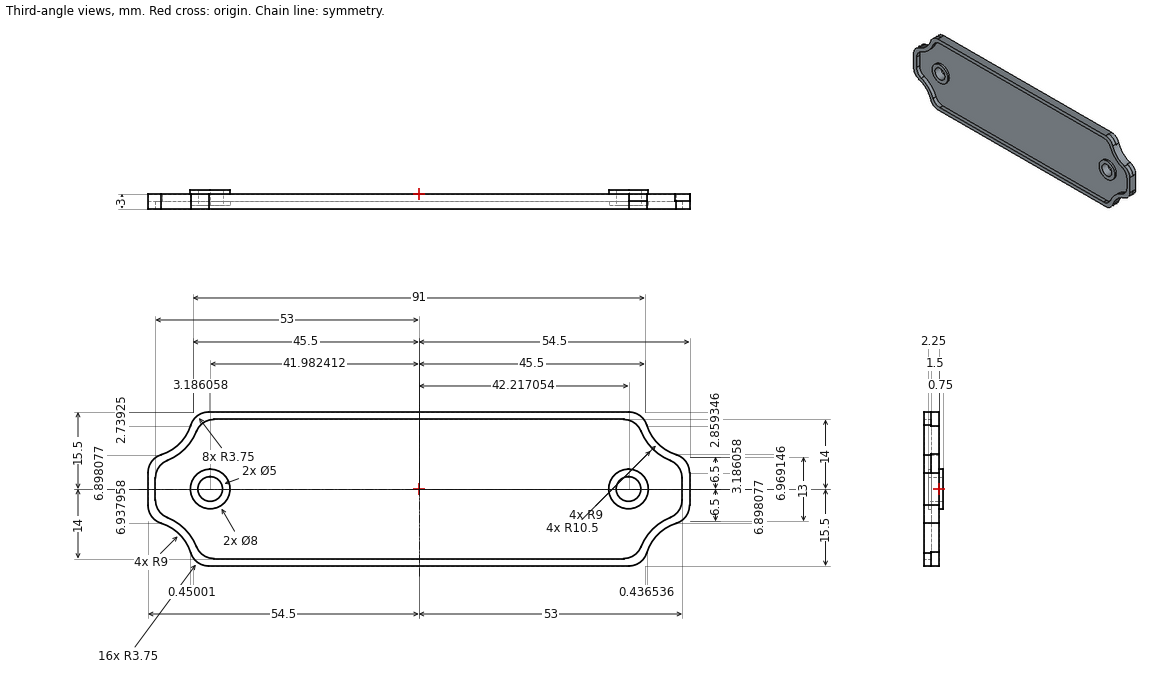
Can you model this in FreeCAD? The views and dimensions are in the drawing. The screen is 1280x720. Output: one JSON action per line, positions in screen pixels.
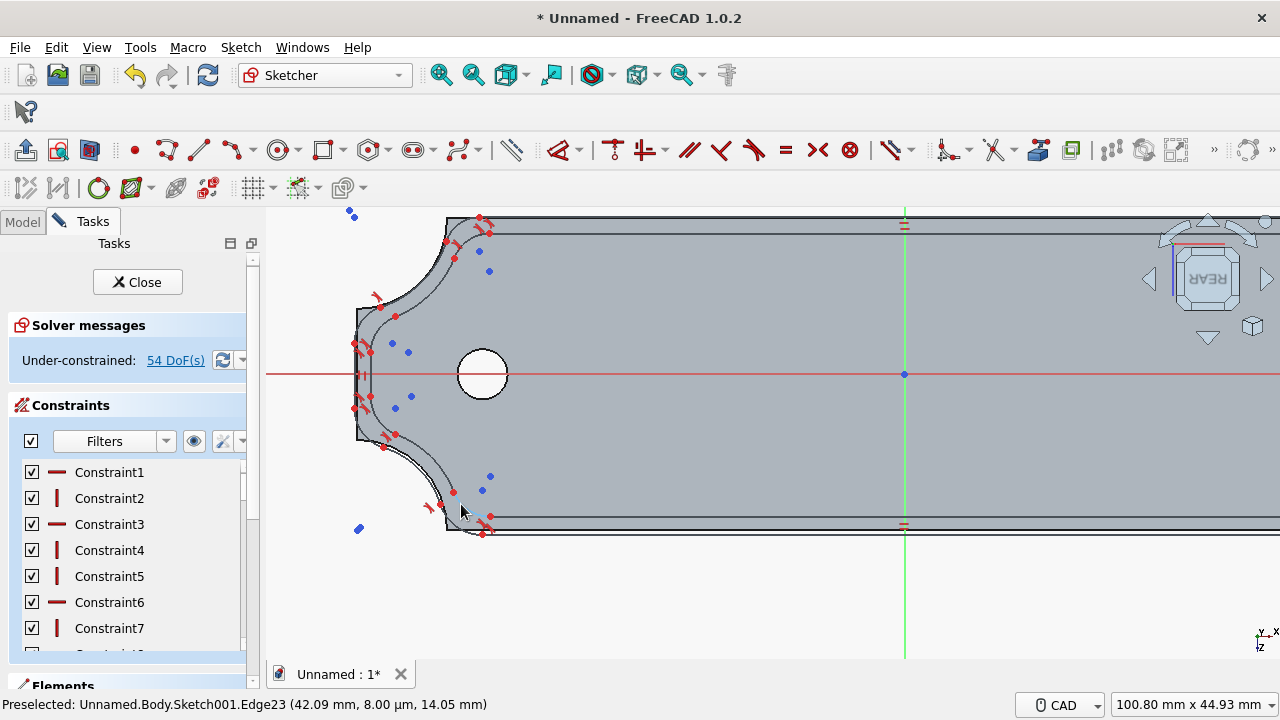
{"action": "left_click", "coordinate": [462, 504]}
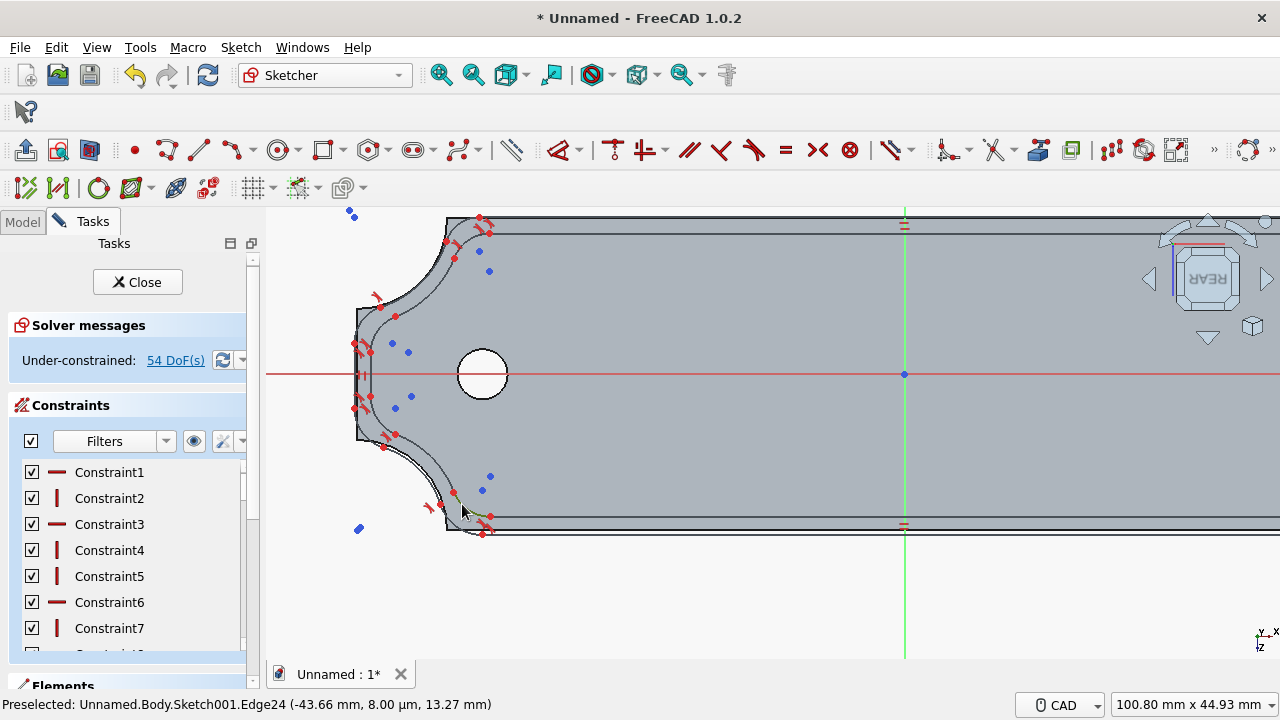
{"action": "left_click", "coordinate": [442, 470]}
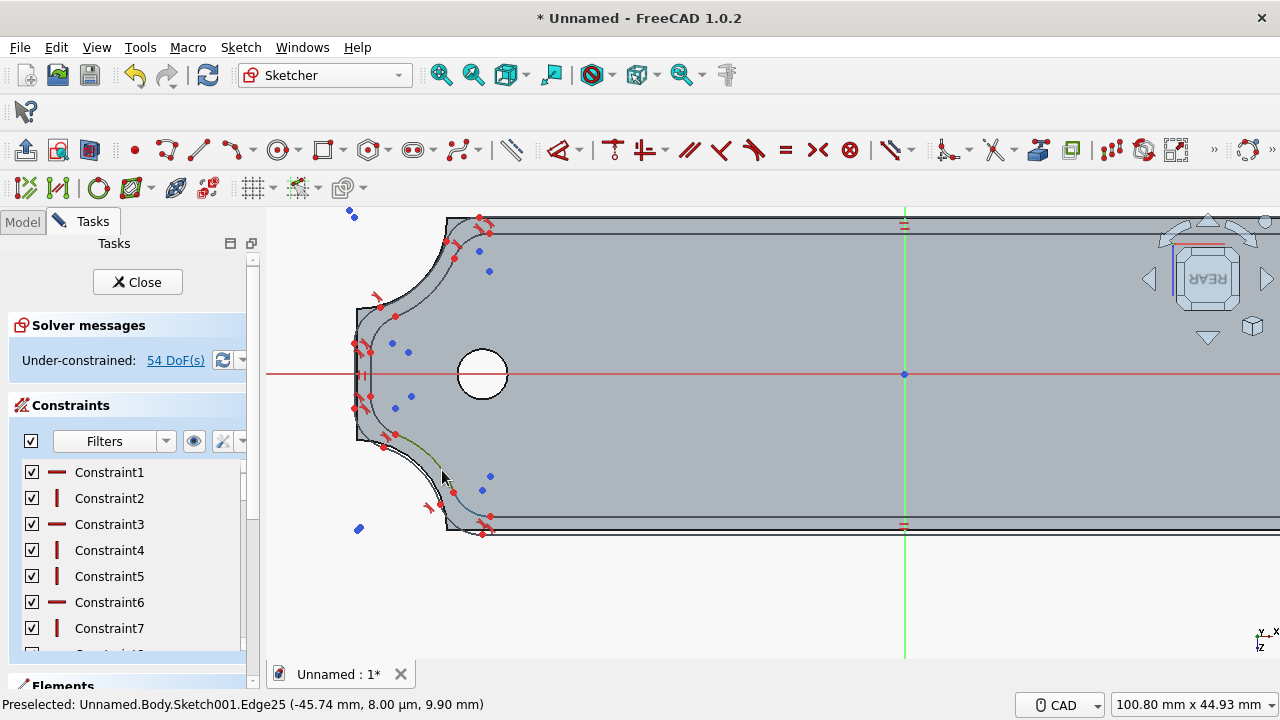
{"action": "left_click", "coordinate": [754, 150]}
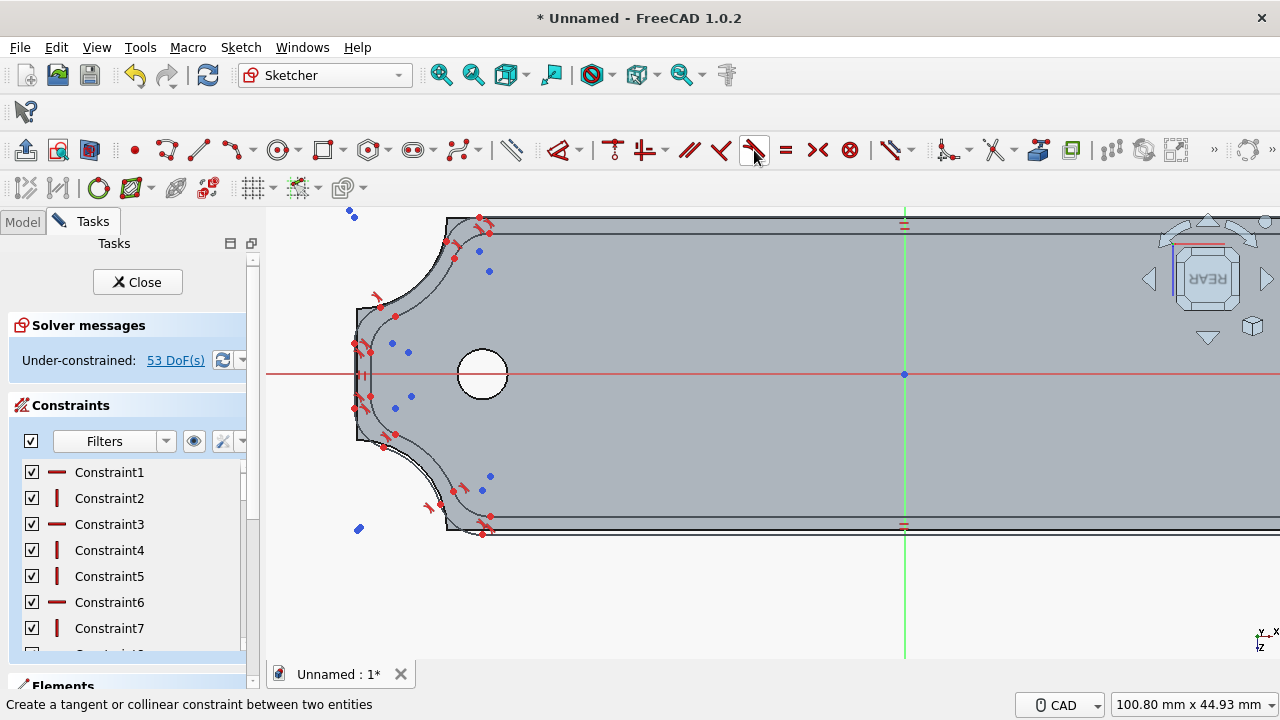
{"action": "left_click", "coordinate": [442, 469]}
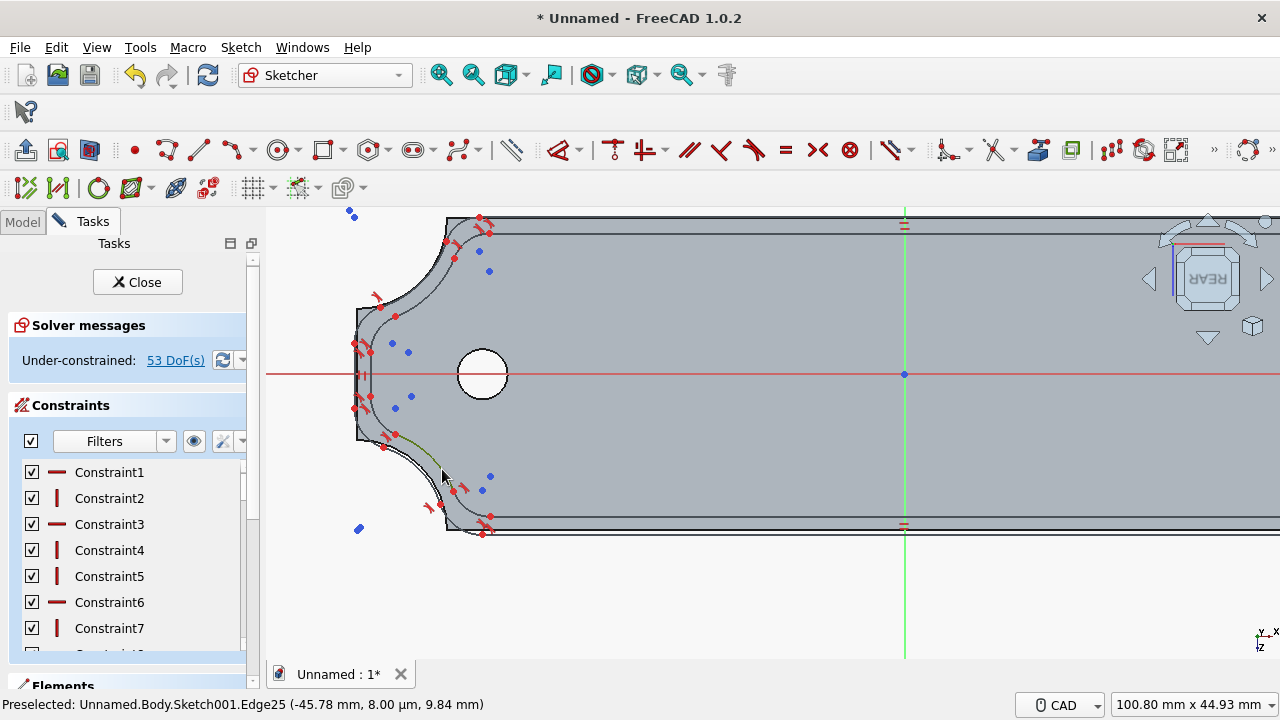
{"action": "left_click", "coordinate": [373, 410]}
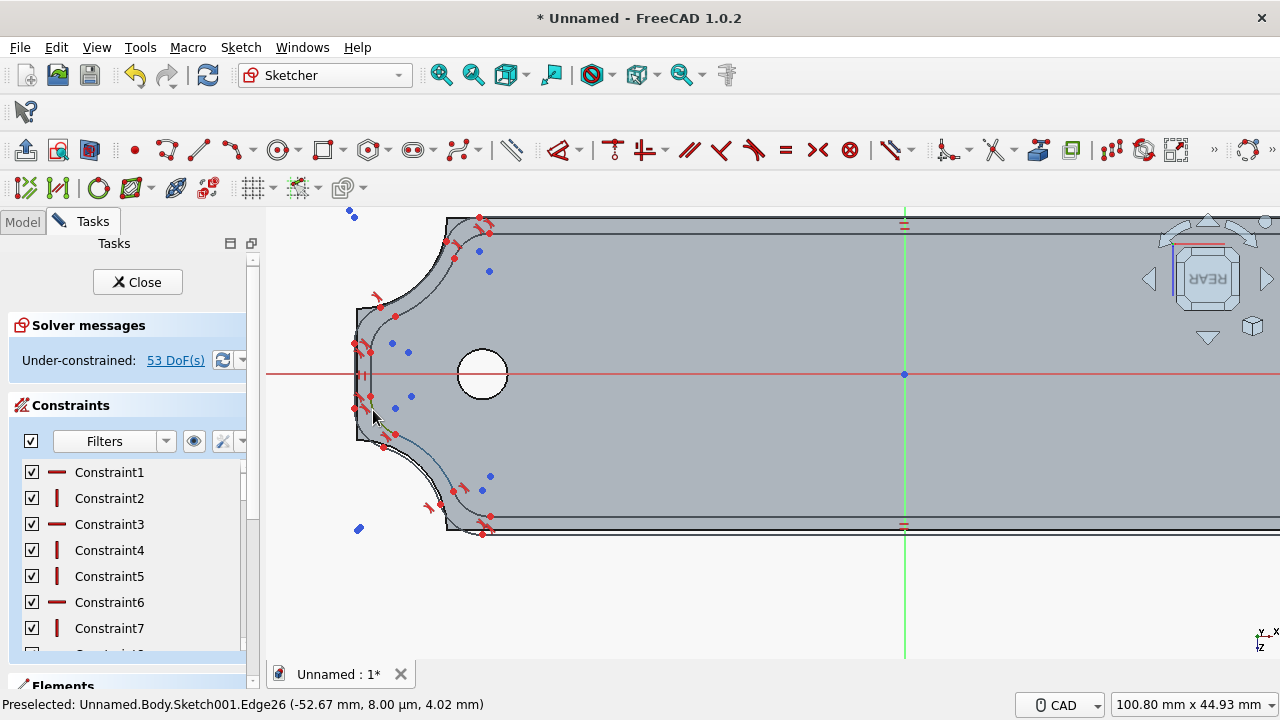
{"action": "left_click", "coordinate": [754, 150]}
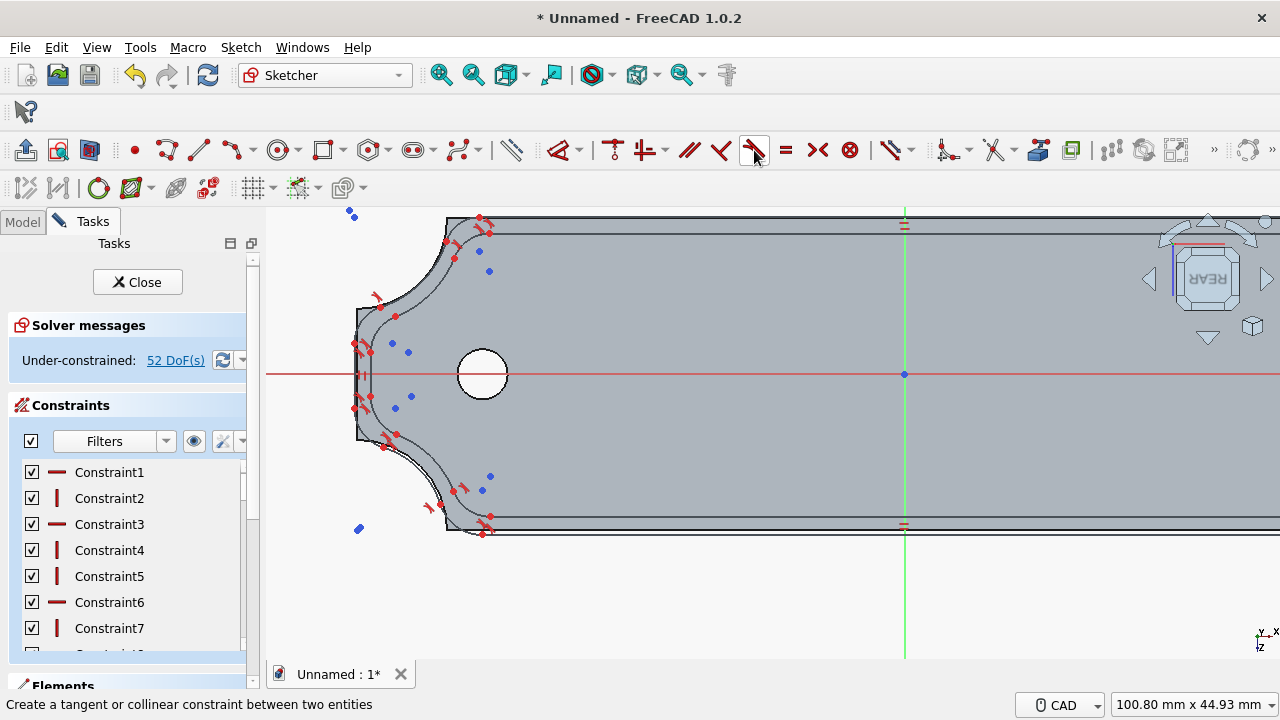
{"action": "left_click", "coordinate": [384, 324]}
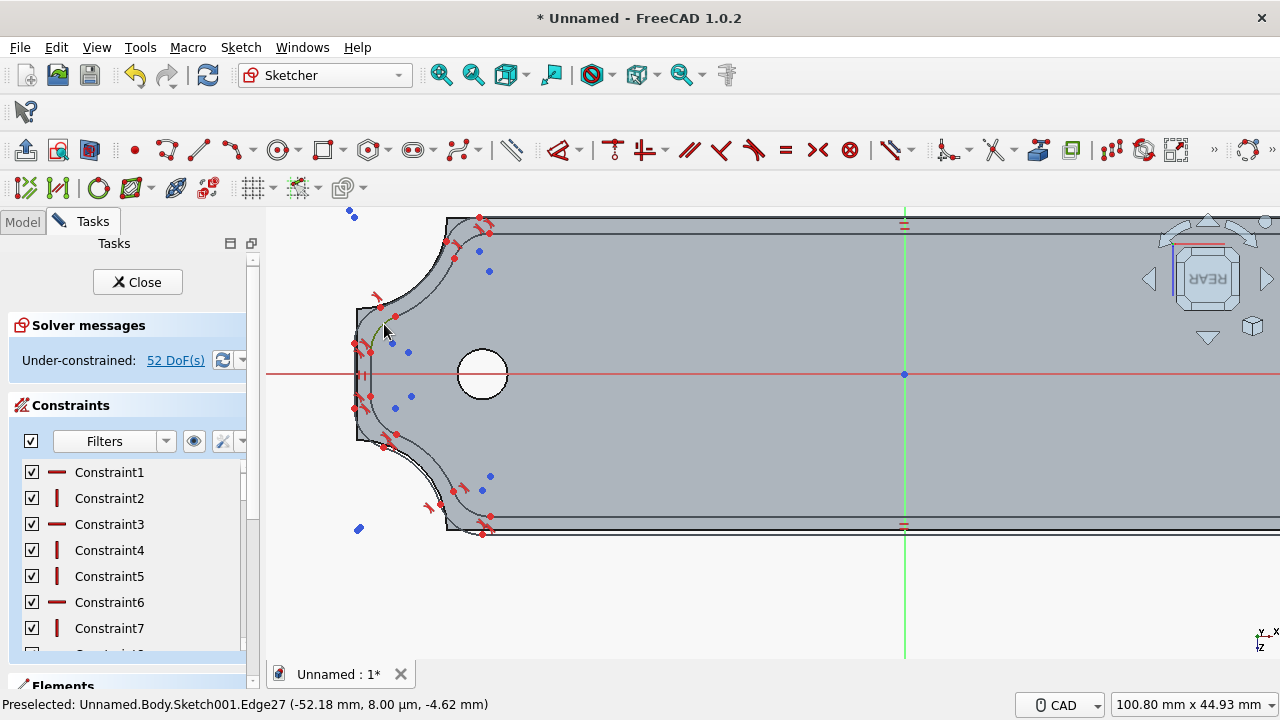
{"action": "left_click", "coordinate": [418, 305]}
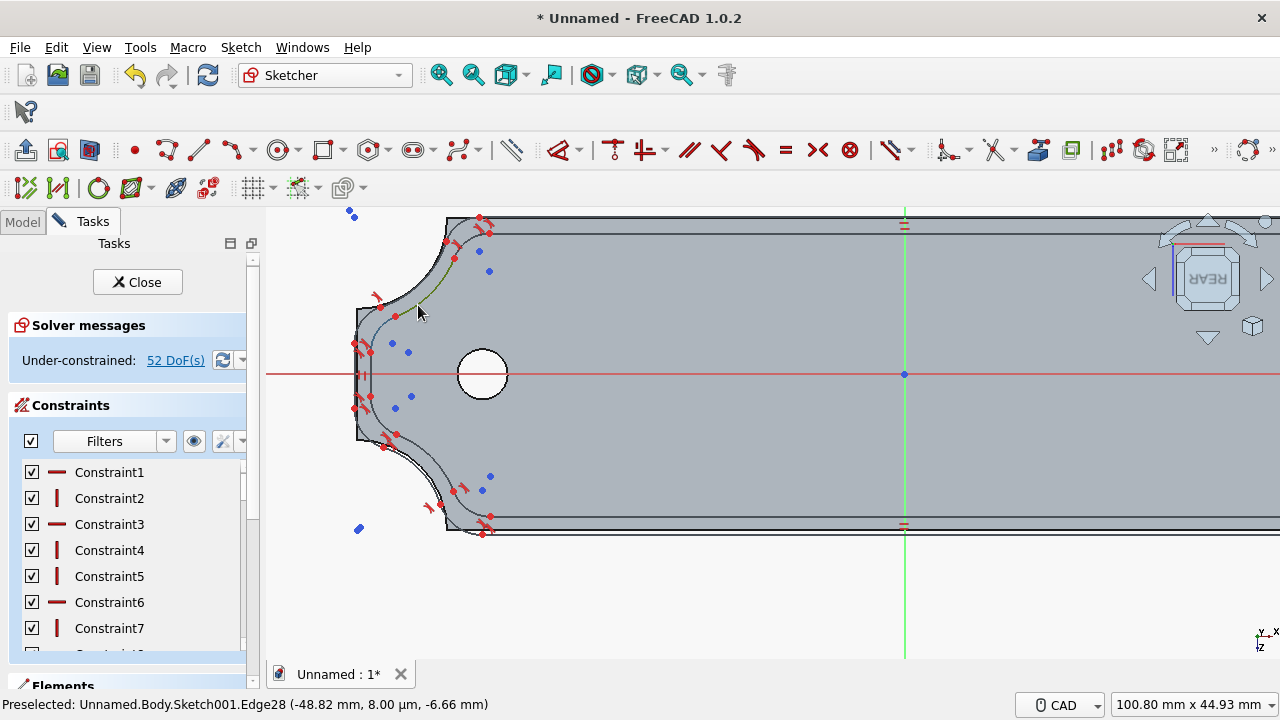
{"action": "left_click", "coordinate": [754, 150]}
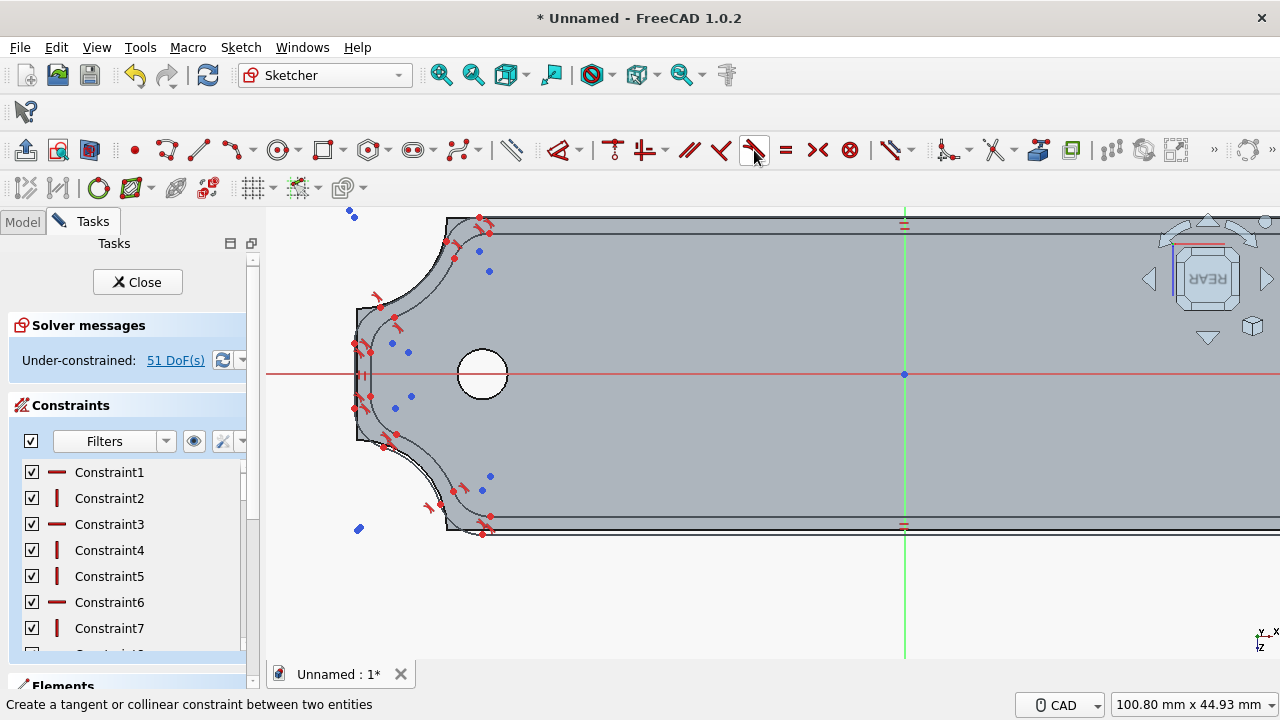
{"action": "left_click", "coordinate": [417, 305]}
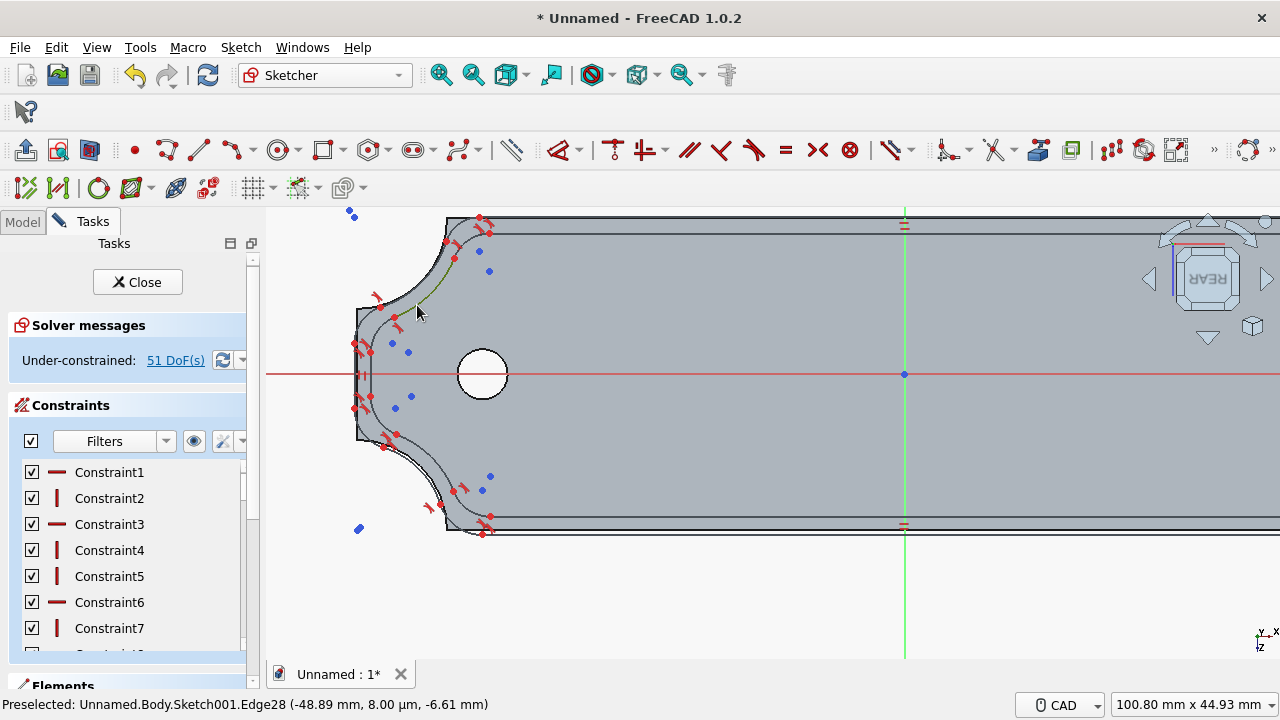
{"action": "left_click", "coordinate": [476, 236]}